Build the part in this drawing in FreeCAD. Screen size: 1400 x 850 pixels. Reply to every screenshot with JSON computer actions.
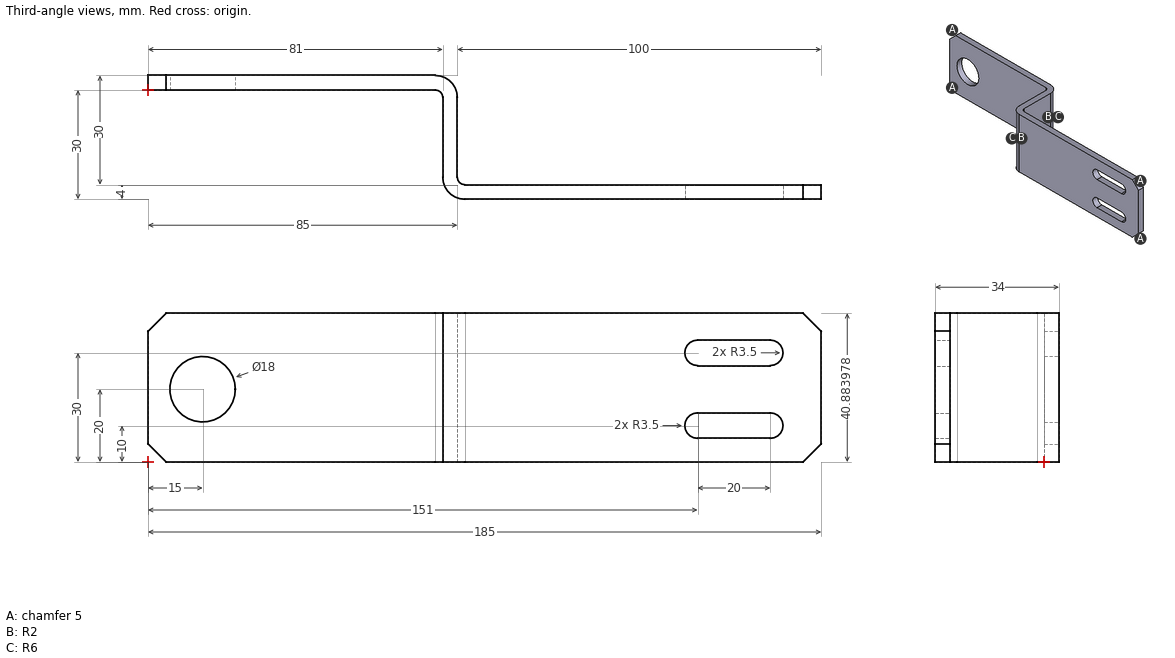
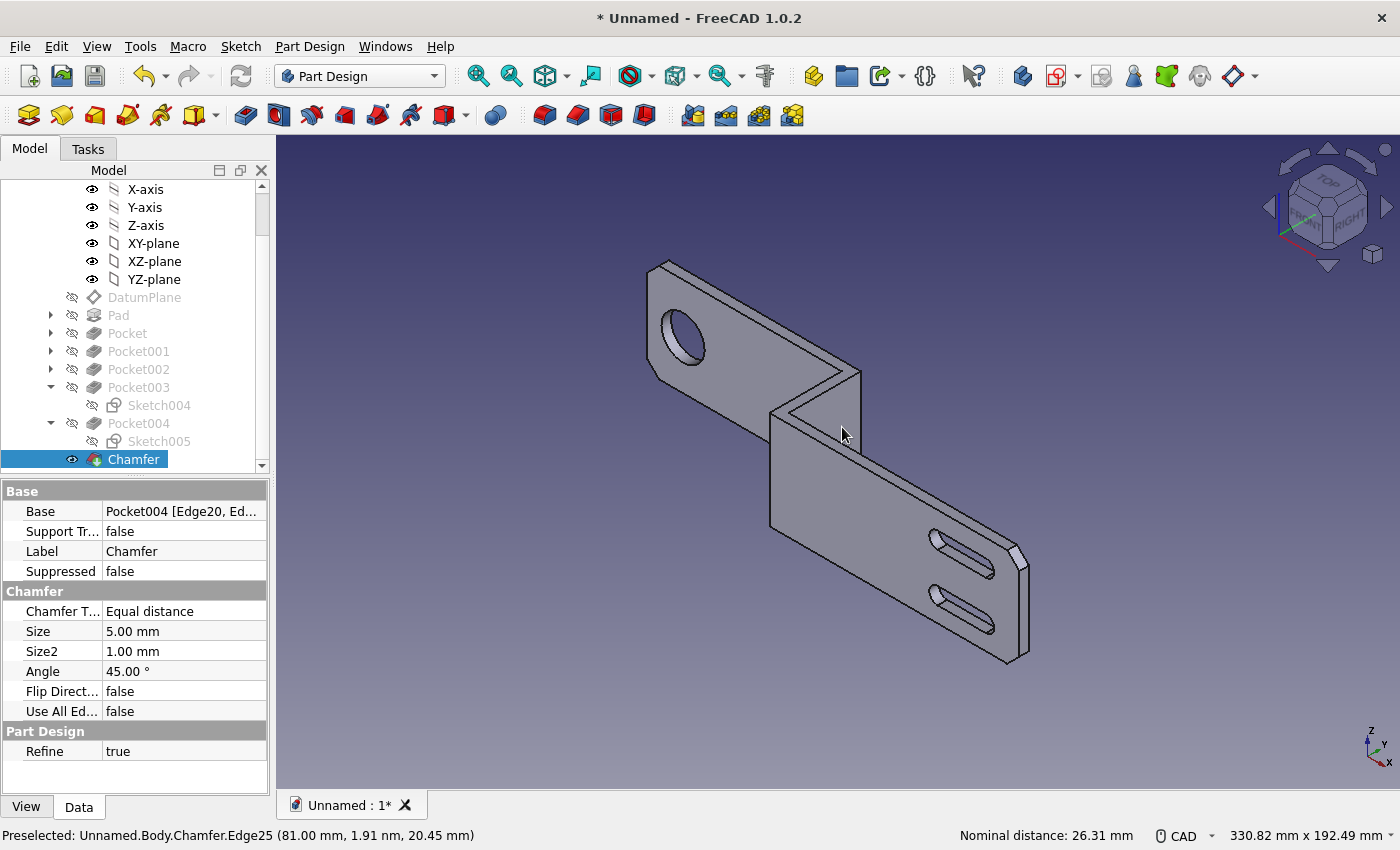
{"action": "left_click", "coordinate": [545, 116]}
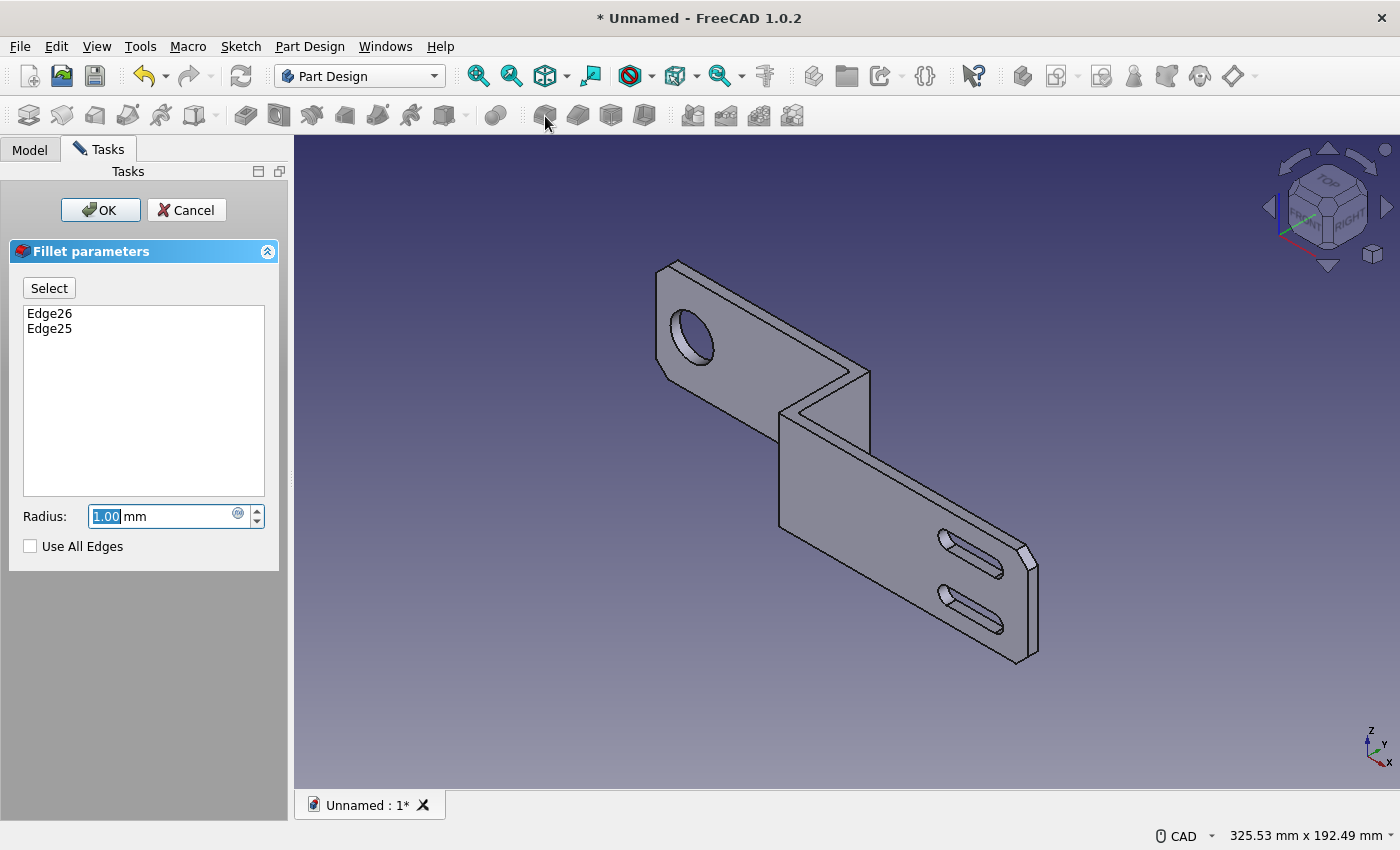
{"action": "type", "text": "2"}
{"action": "key", "text": "Tab"}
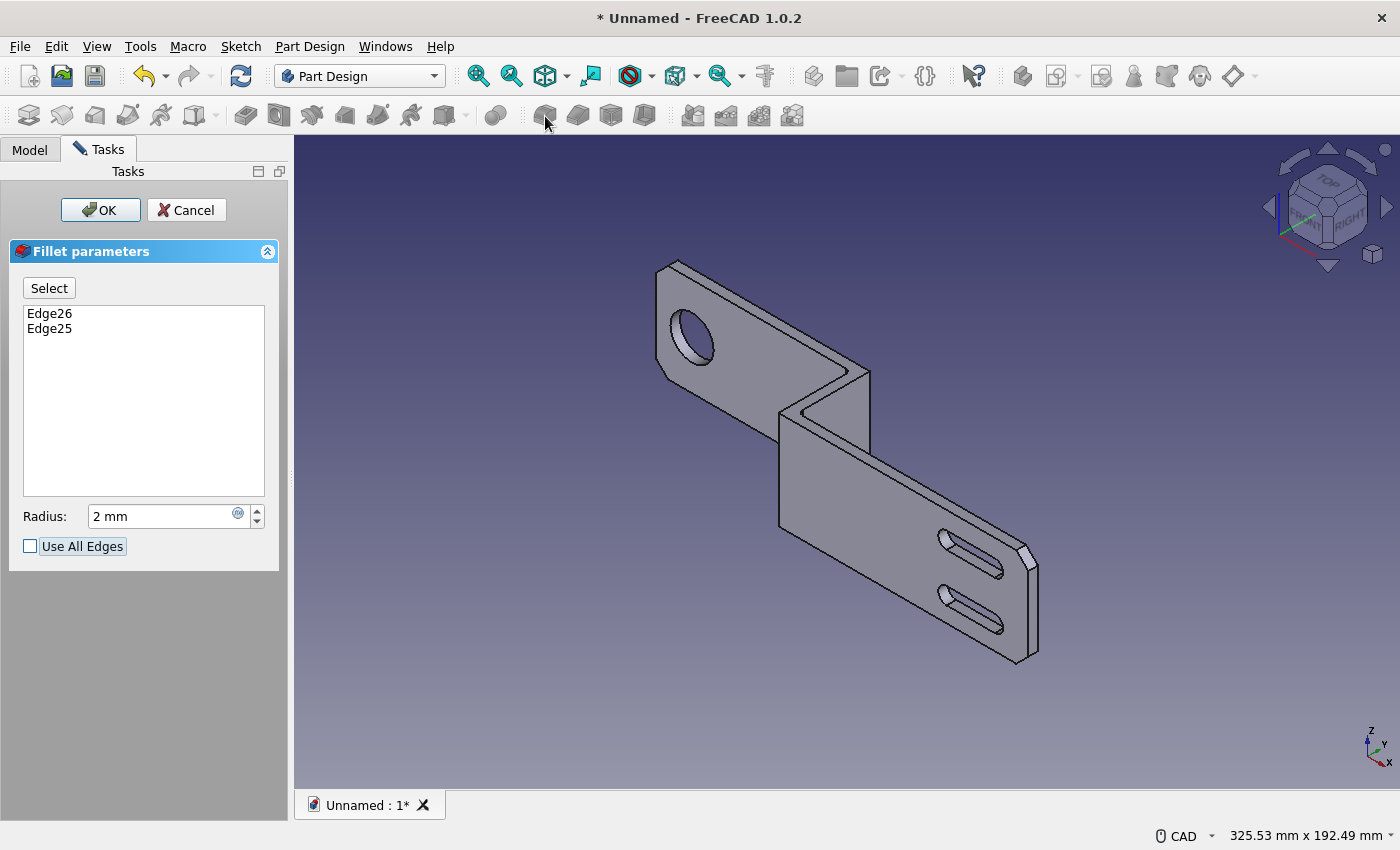
{"action": "left_click", "coordinate": [101, 210]}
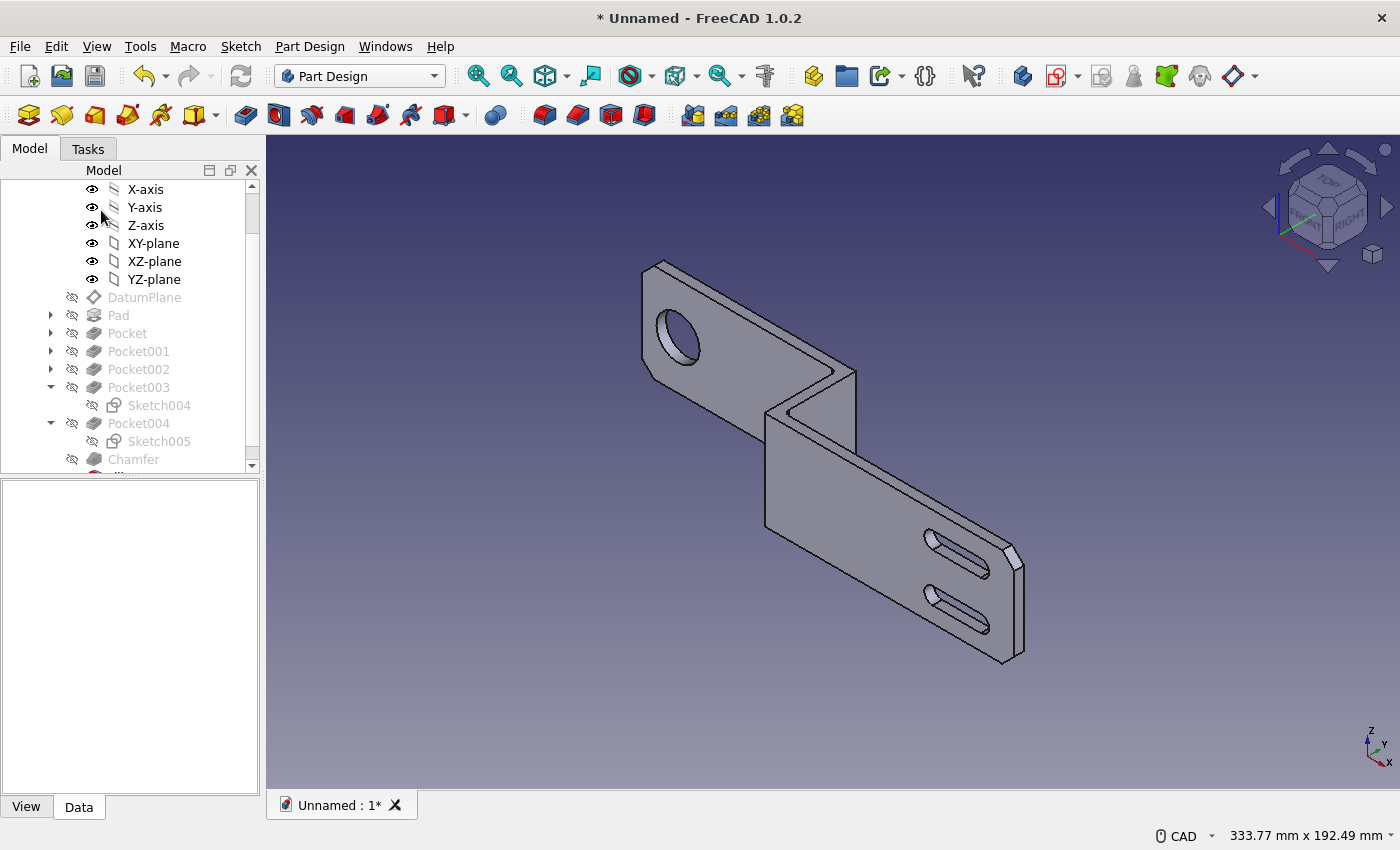
{"action": "key", "text": "2"}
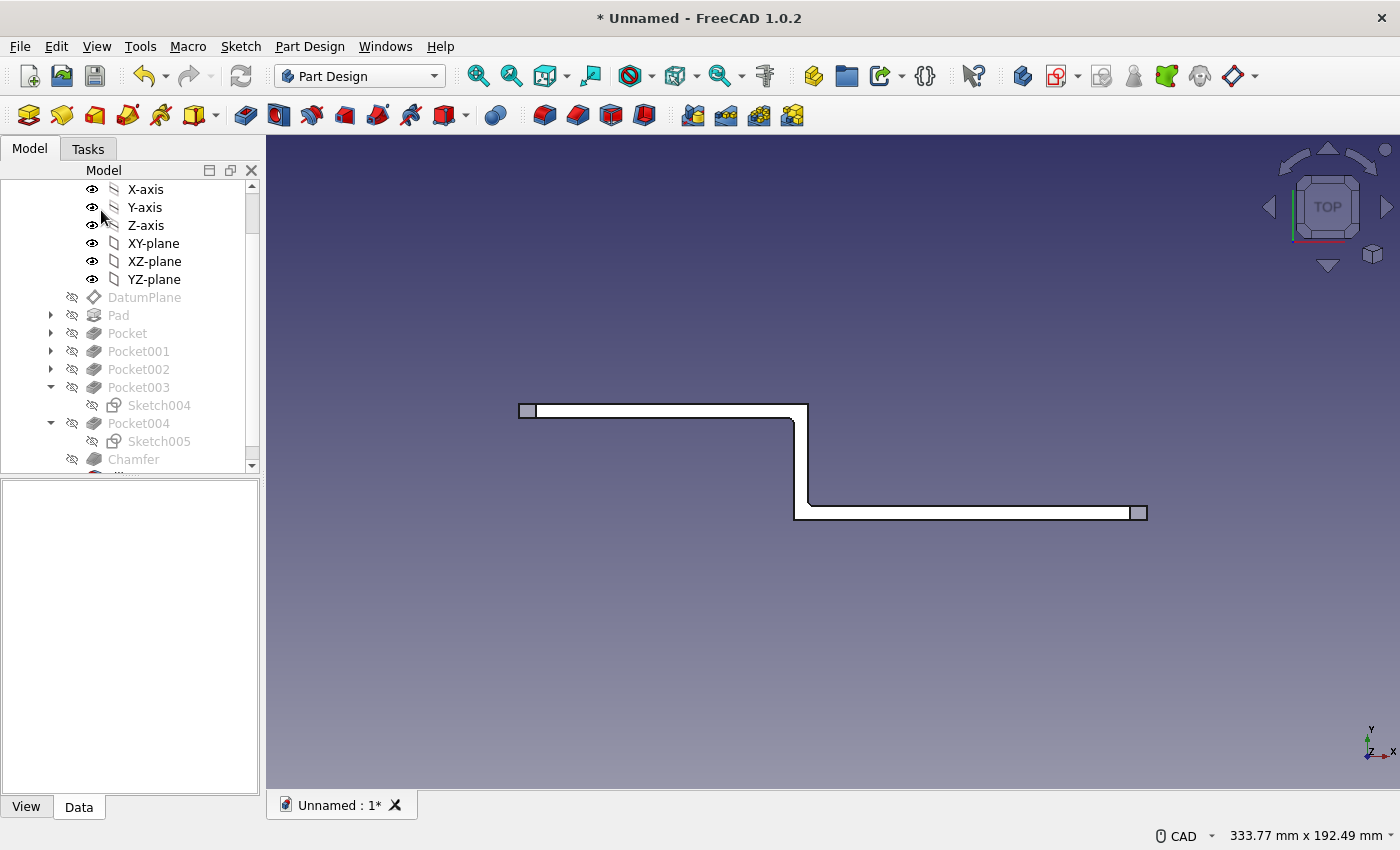
{"action": "key", "text": "0"}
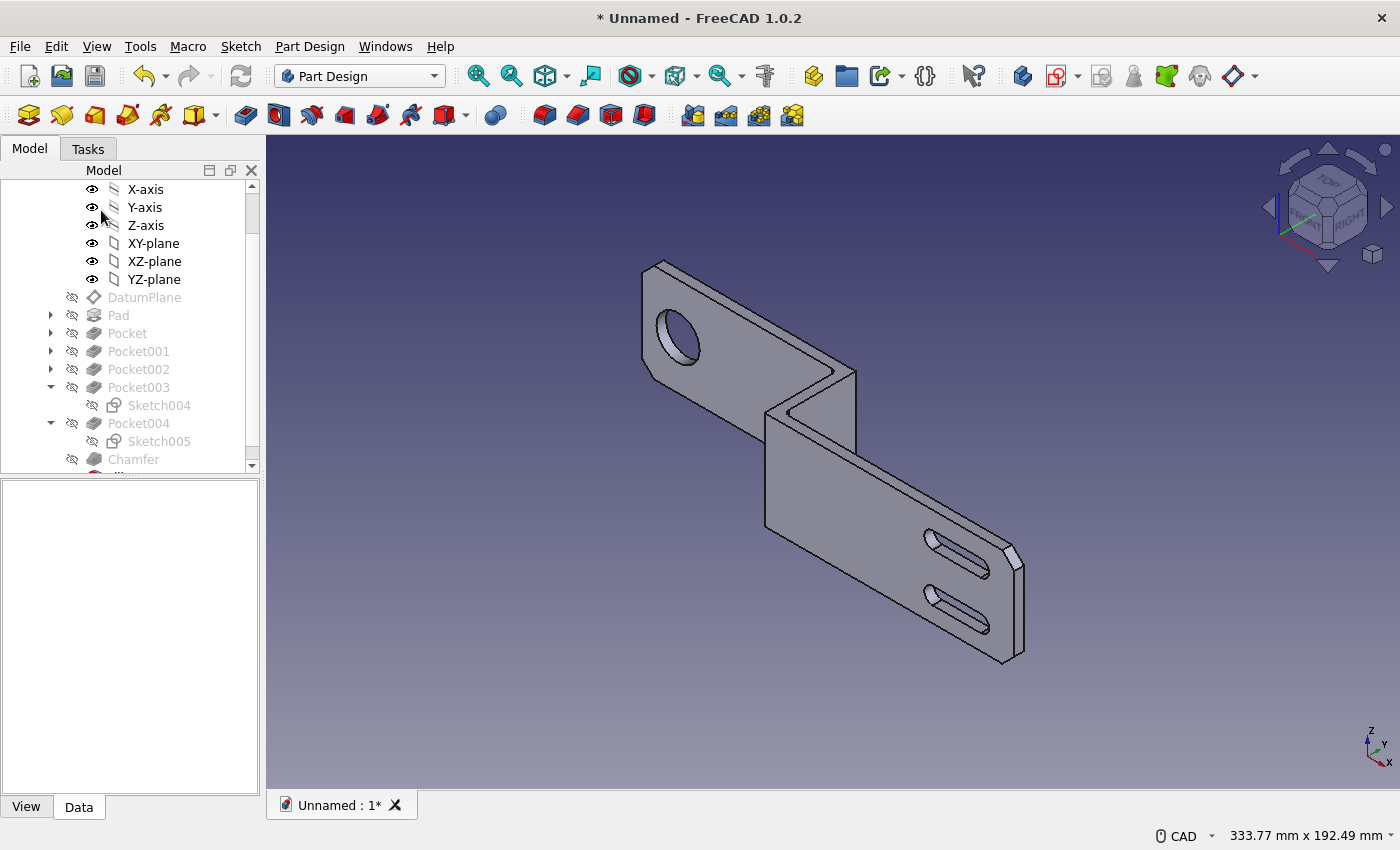
{"action": "key", "text": "1"}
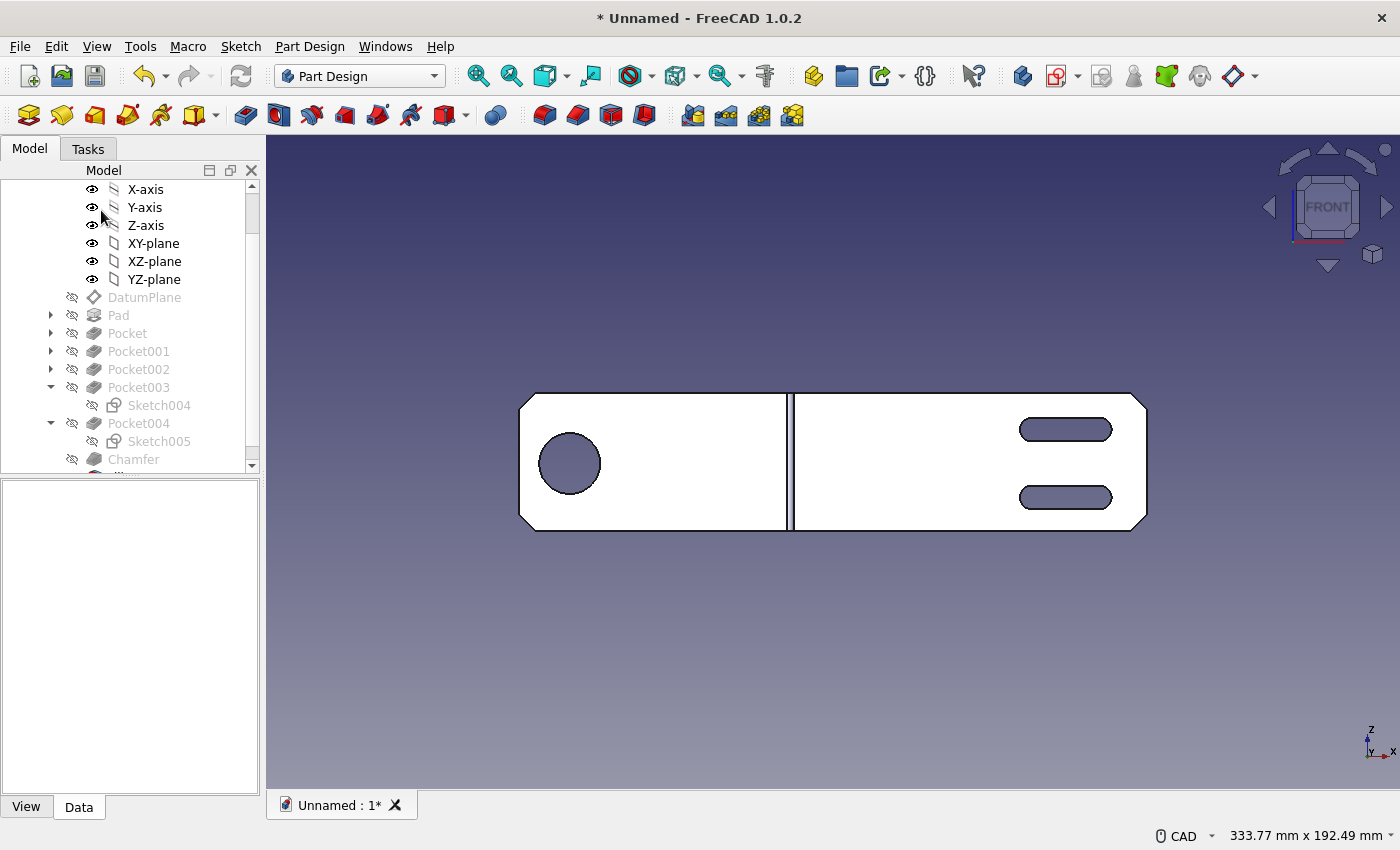
{"action": "left_click", "coordinate": [794, 461]}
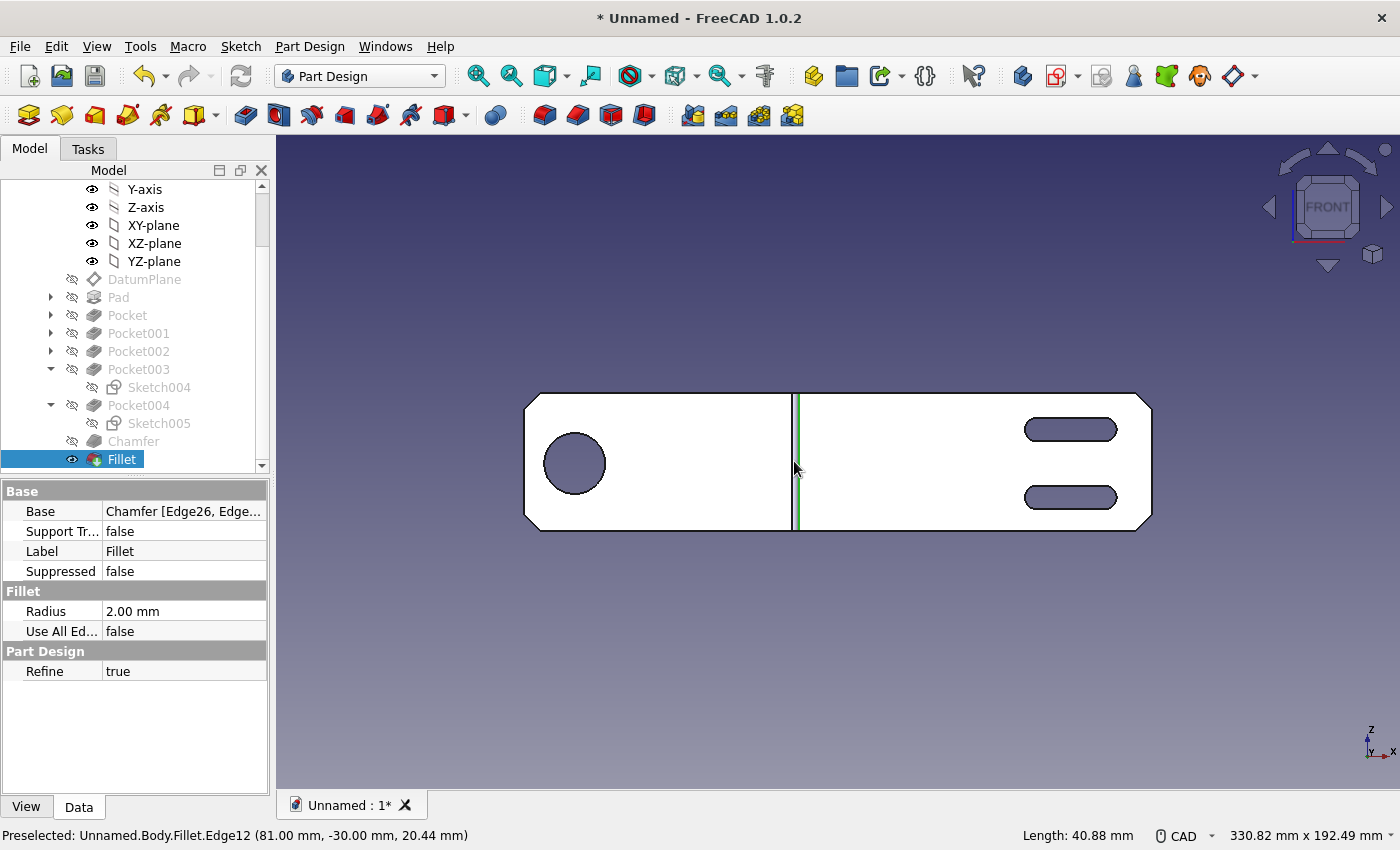
{"action": "key", "text": "3"}